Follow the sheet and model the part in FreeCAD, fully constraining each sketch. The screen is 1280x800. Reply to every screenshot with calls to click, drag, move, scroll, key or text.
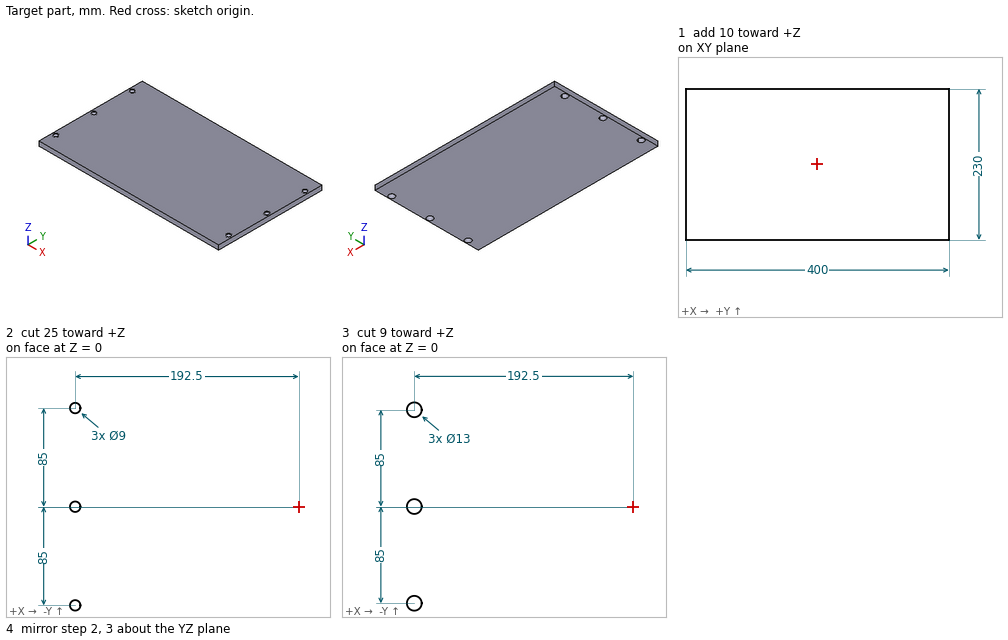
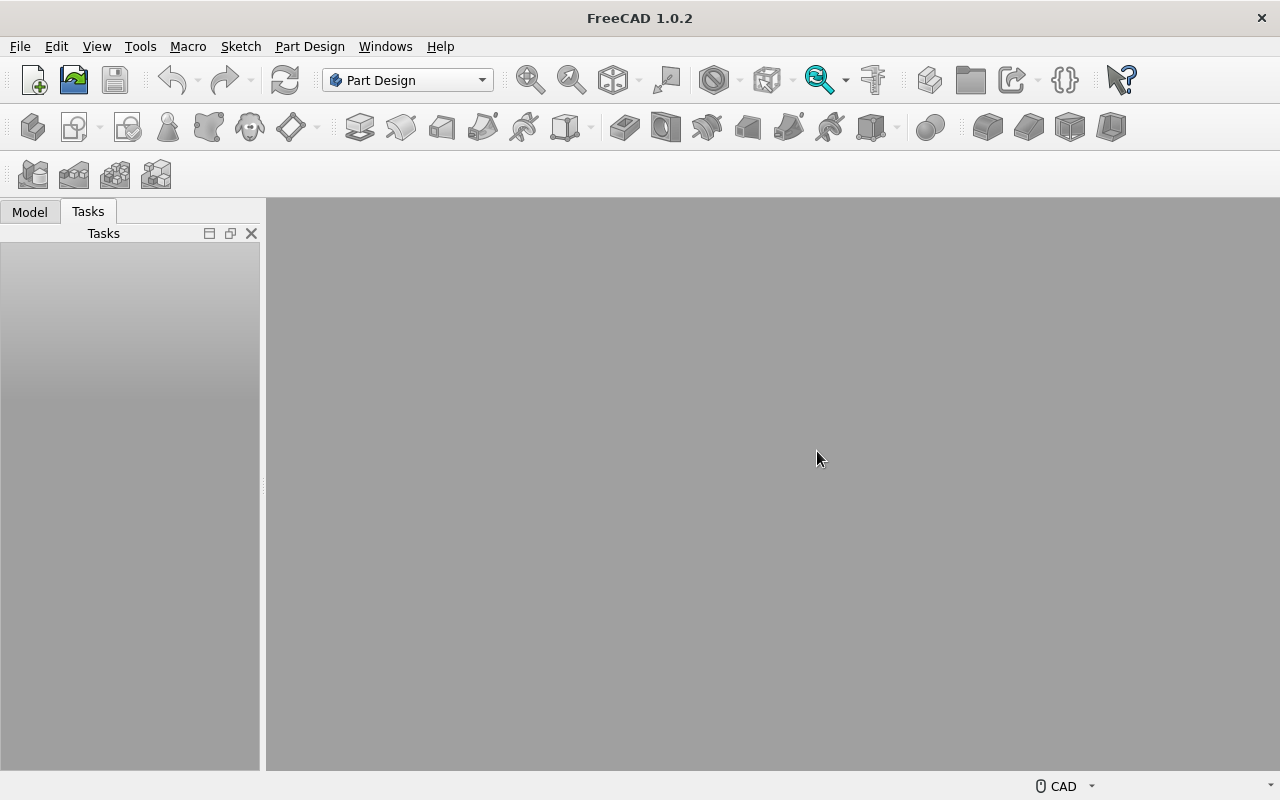
click(33, 80)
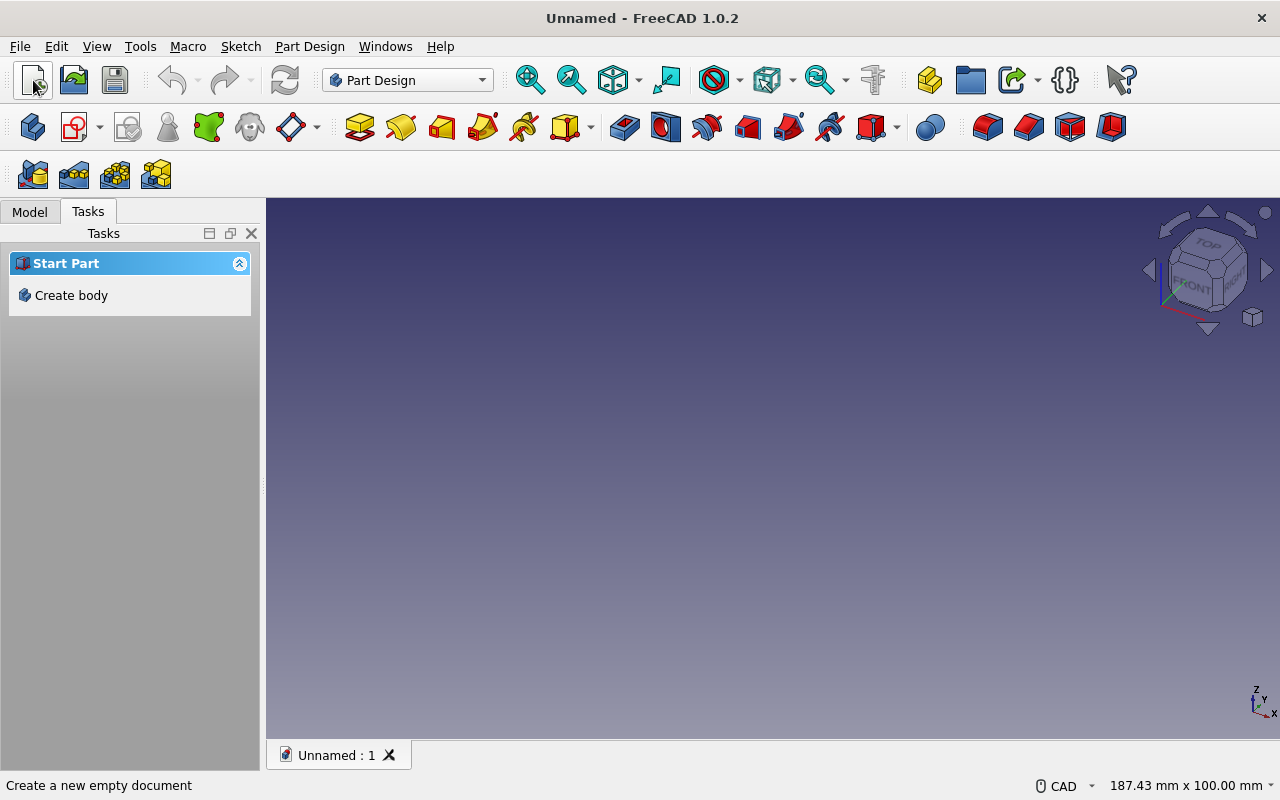
click(74, 128)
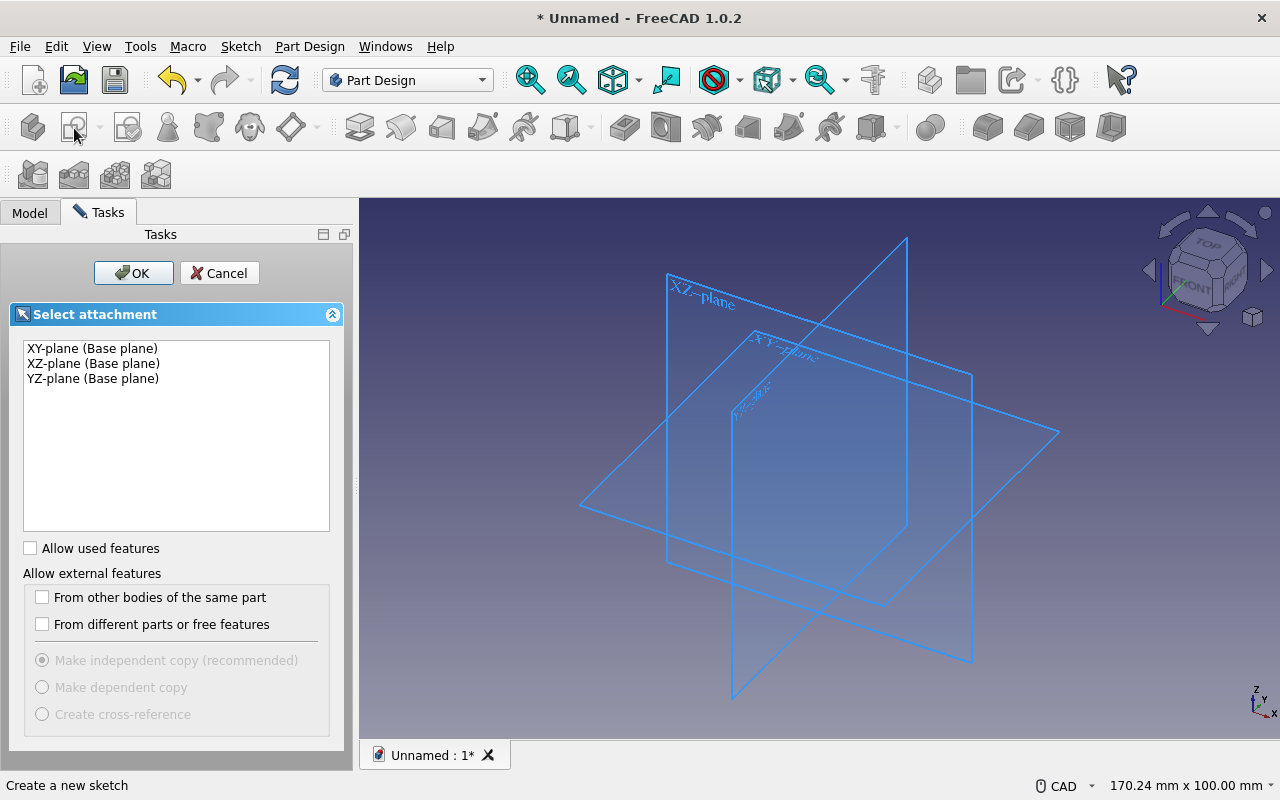
click(84, 348)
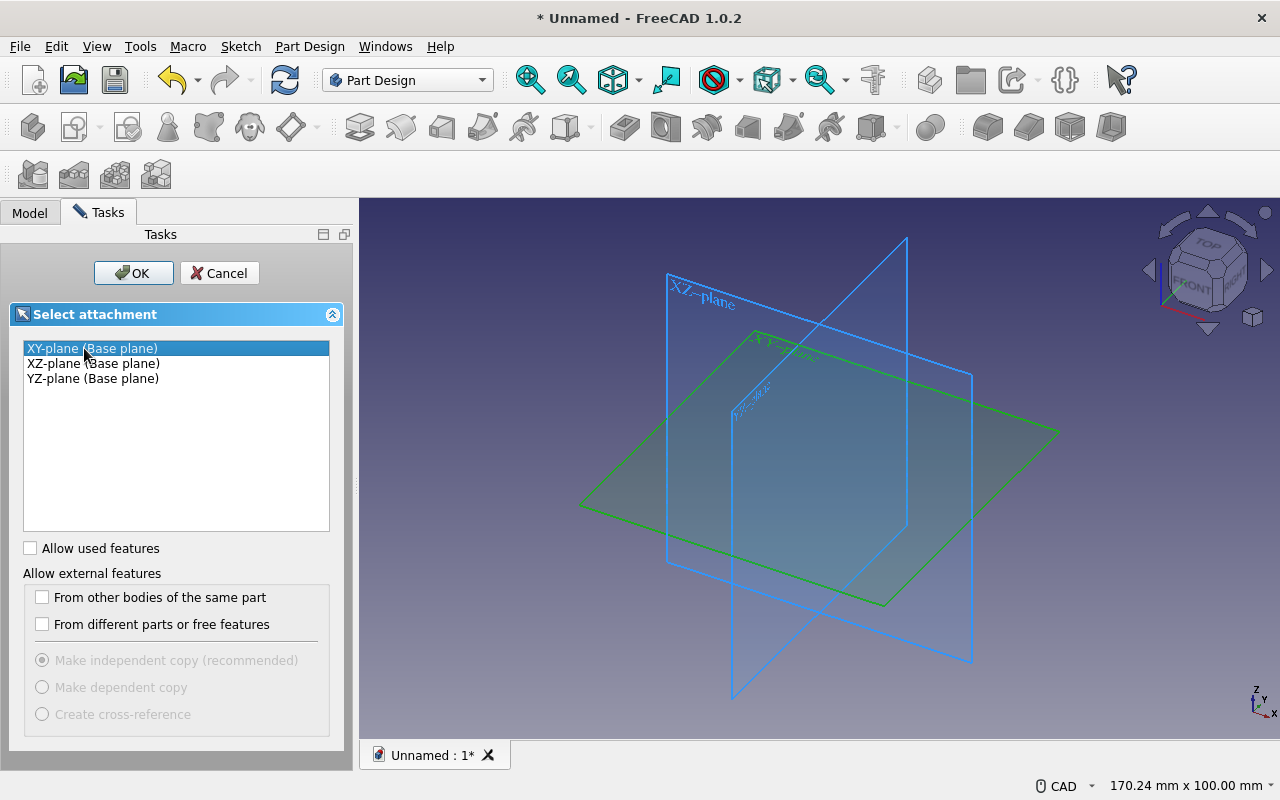
click(134, 273)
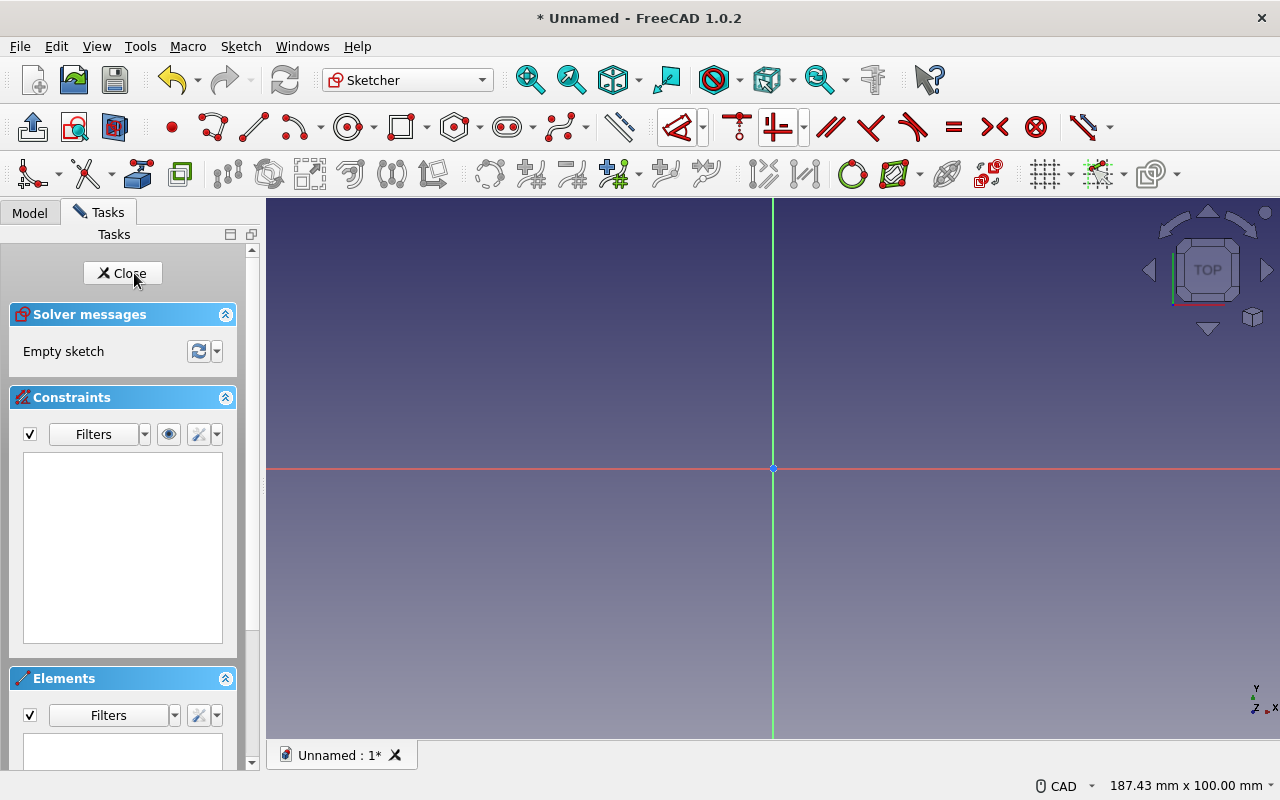
scroll(682, 469, down, 7)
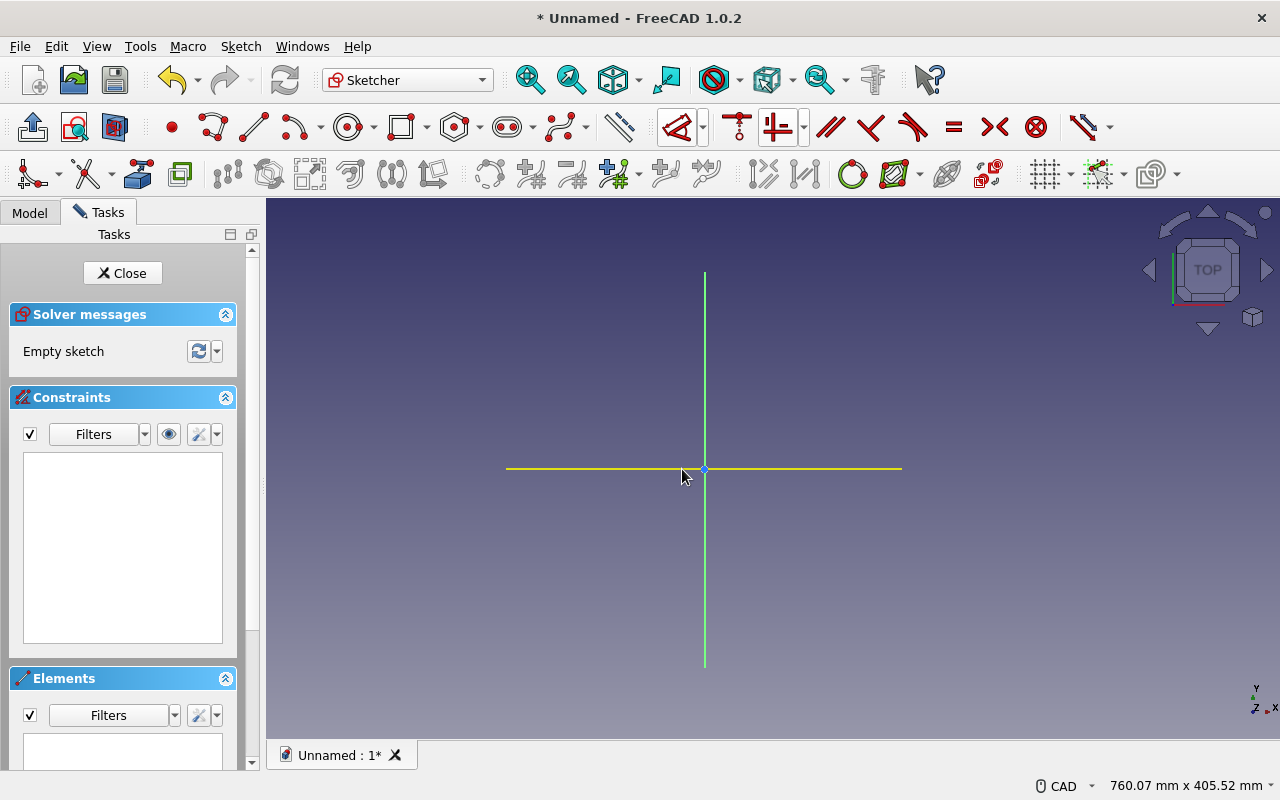
key(g)
key(v)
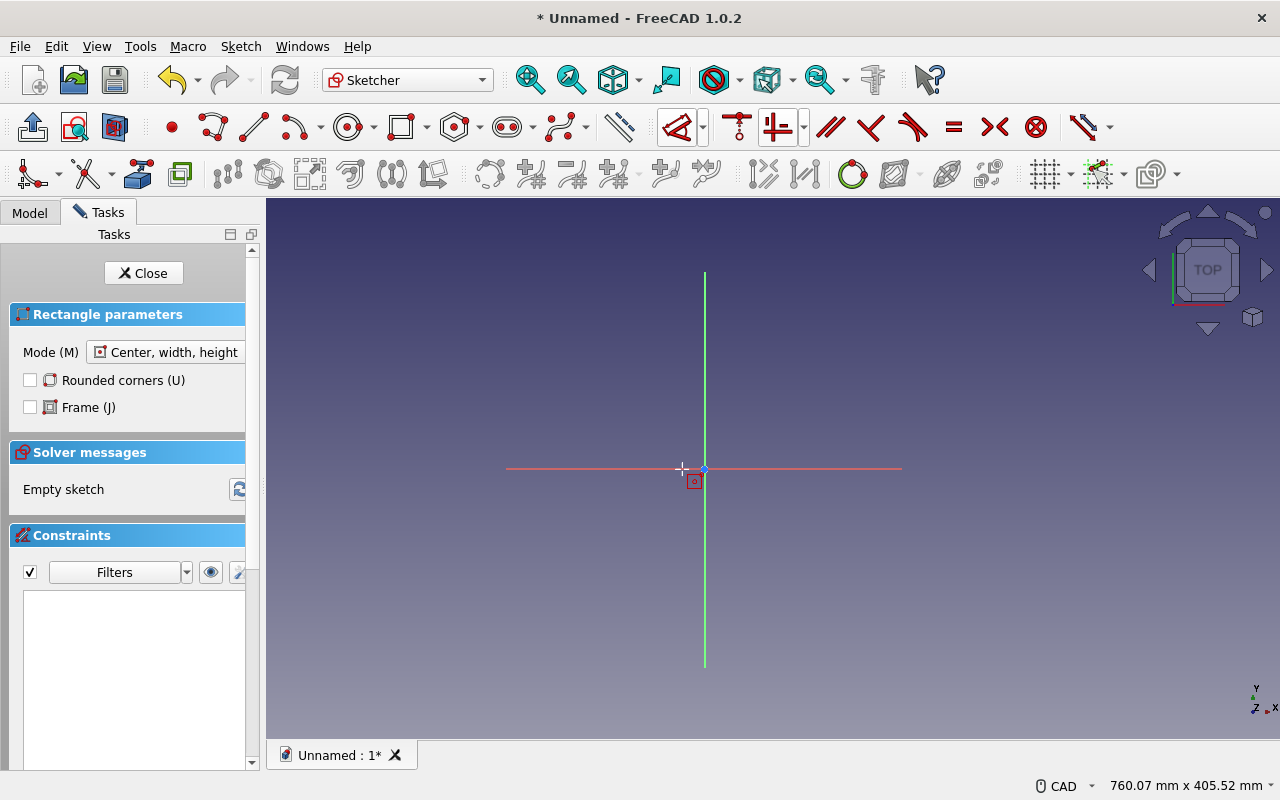
click(705, 469)
move(972, 316)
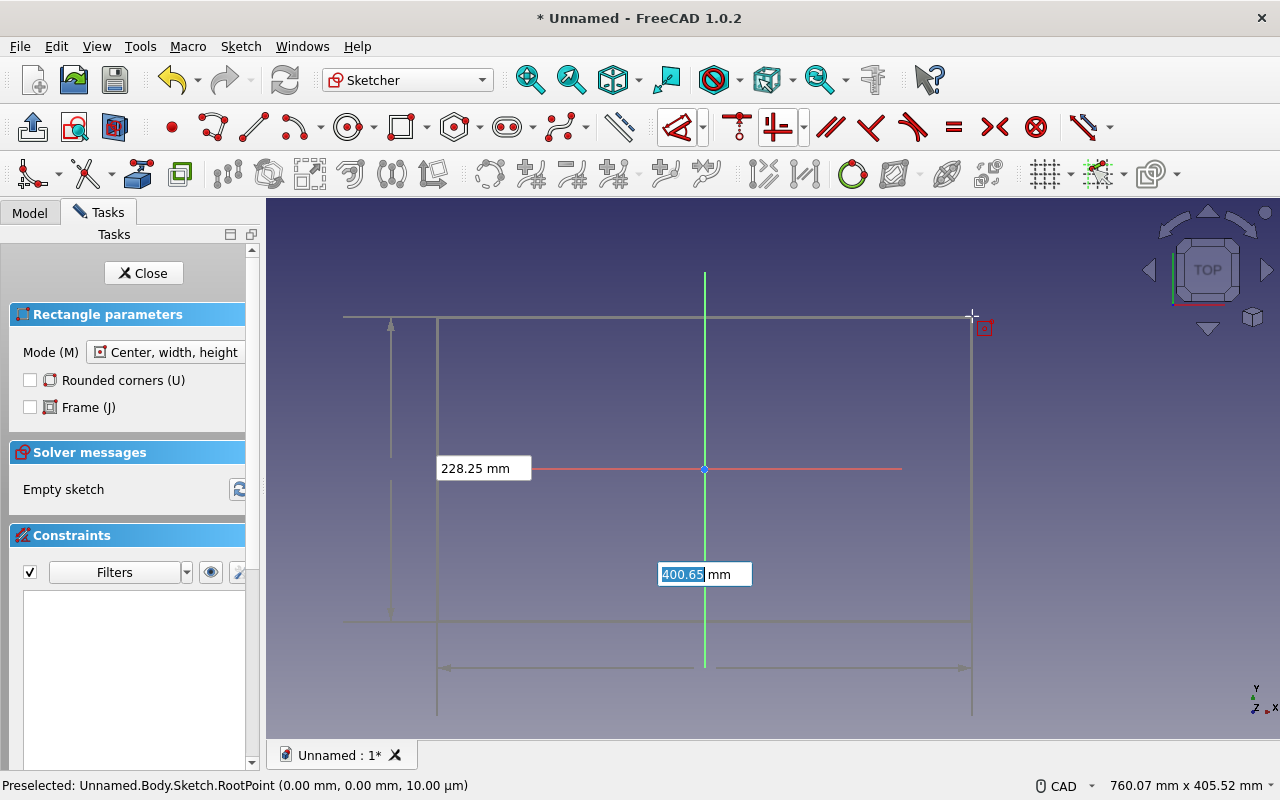
text(400)
key(Tab)
text(230)
key(Return)
key(Escape)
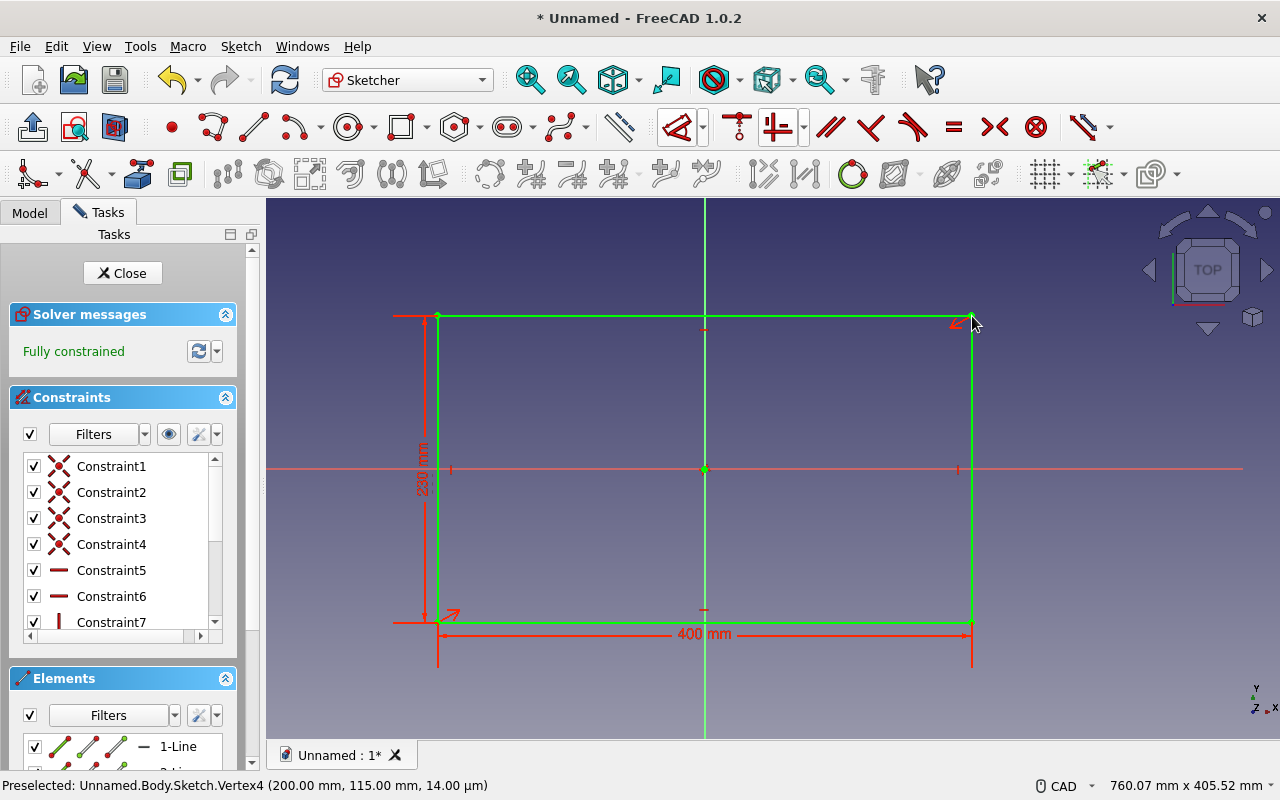
click(123, 273)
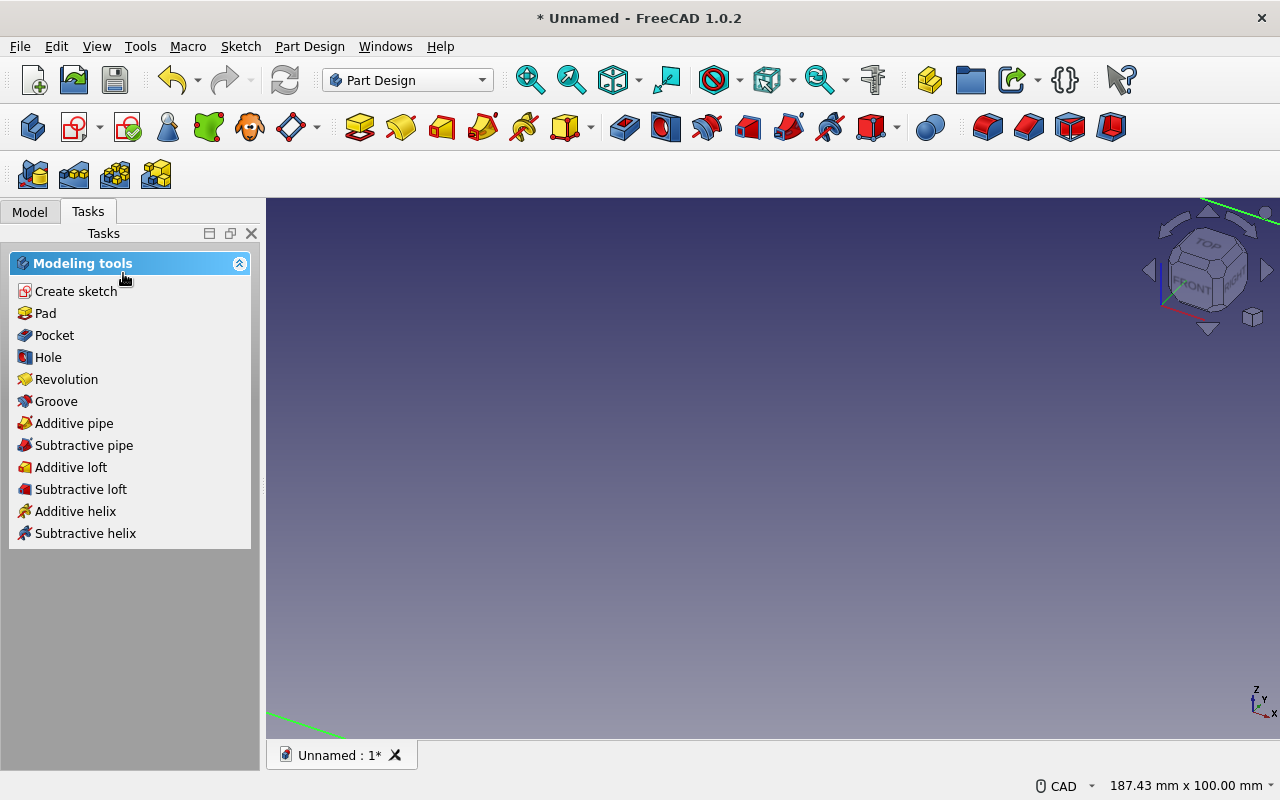
click(360, 128)